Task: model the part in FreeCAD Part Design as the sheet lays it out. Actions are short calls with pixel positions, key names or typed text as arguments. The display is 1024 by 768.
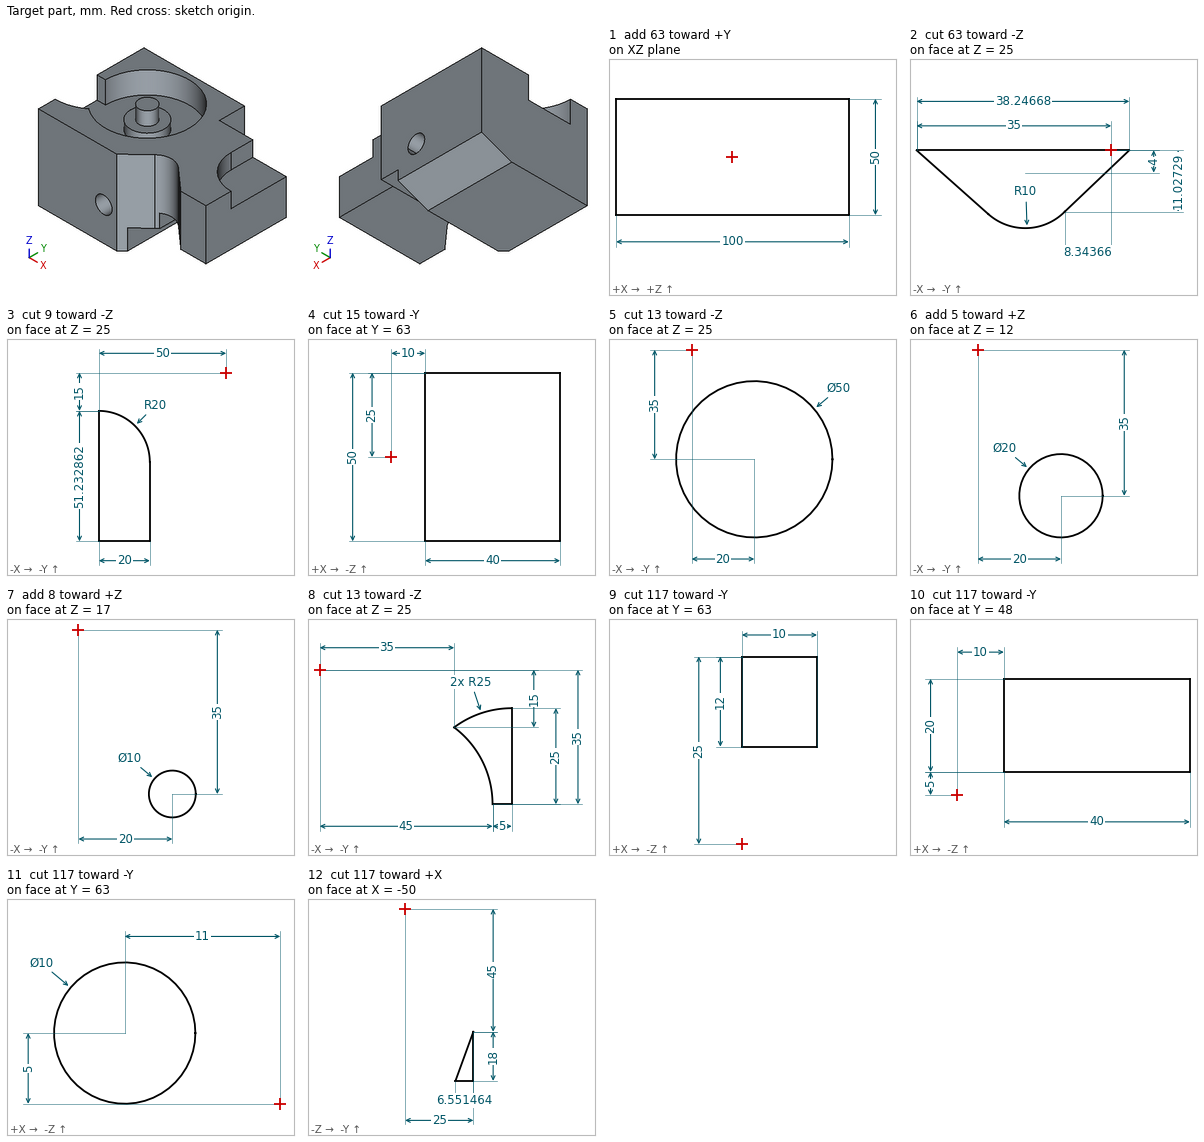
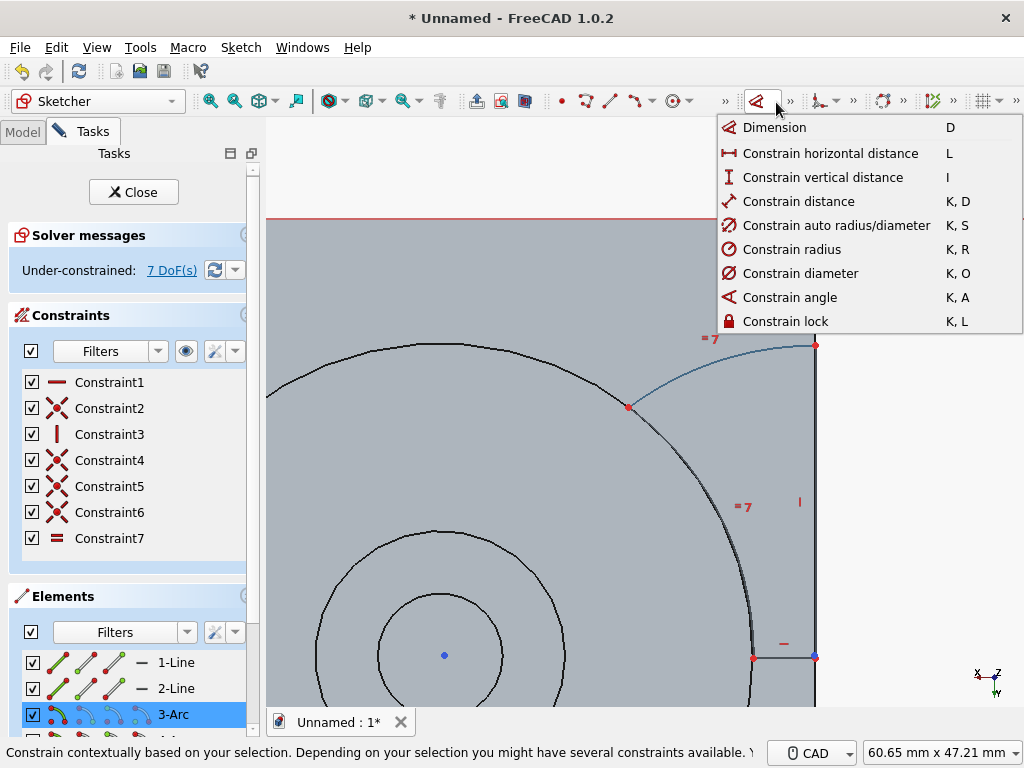
click(870, 249)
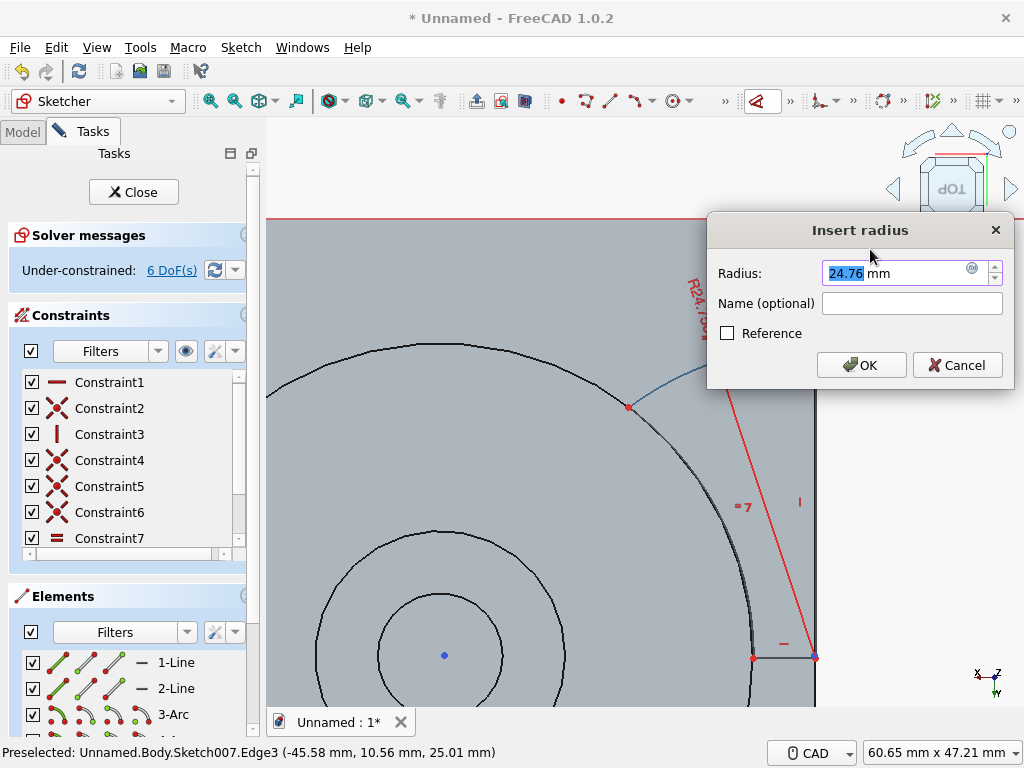
text(25)
key(Return)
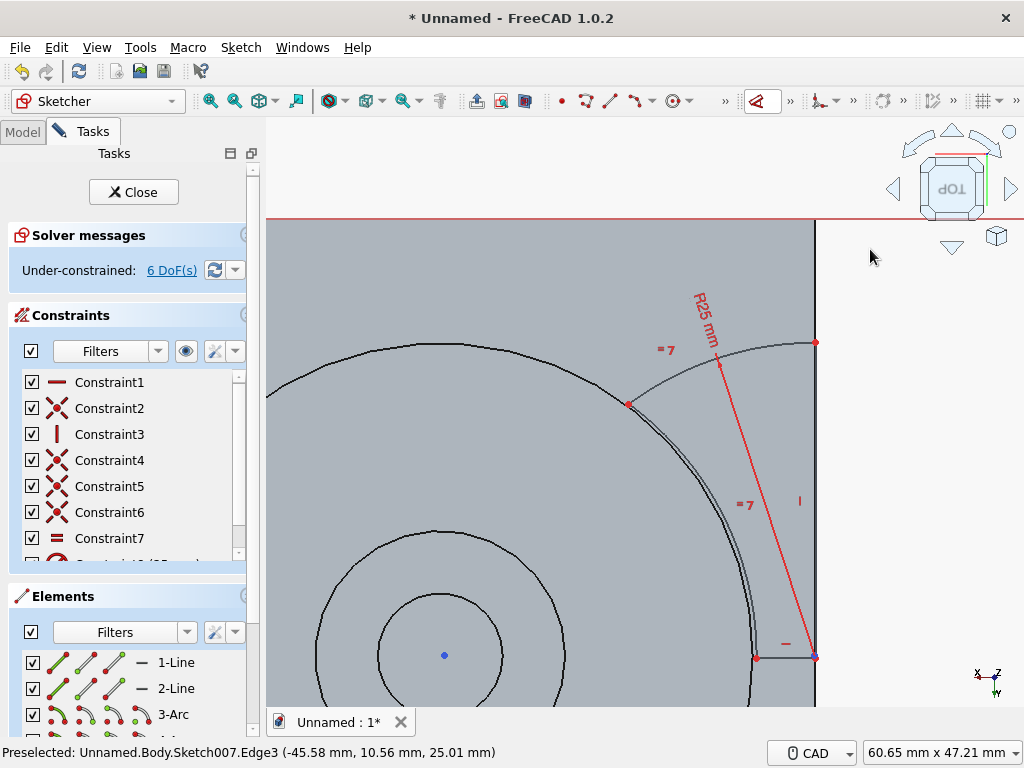
click(774, 658)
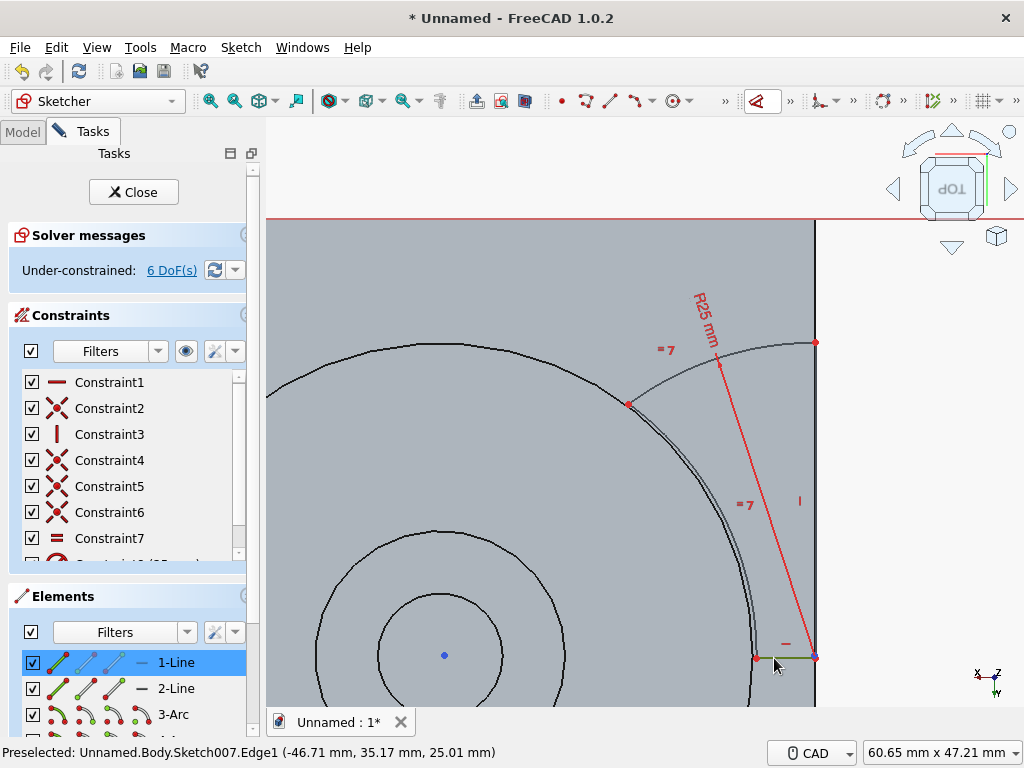
key(l)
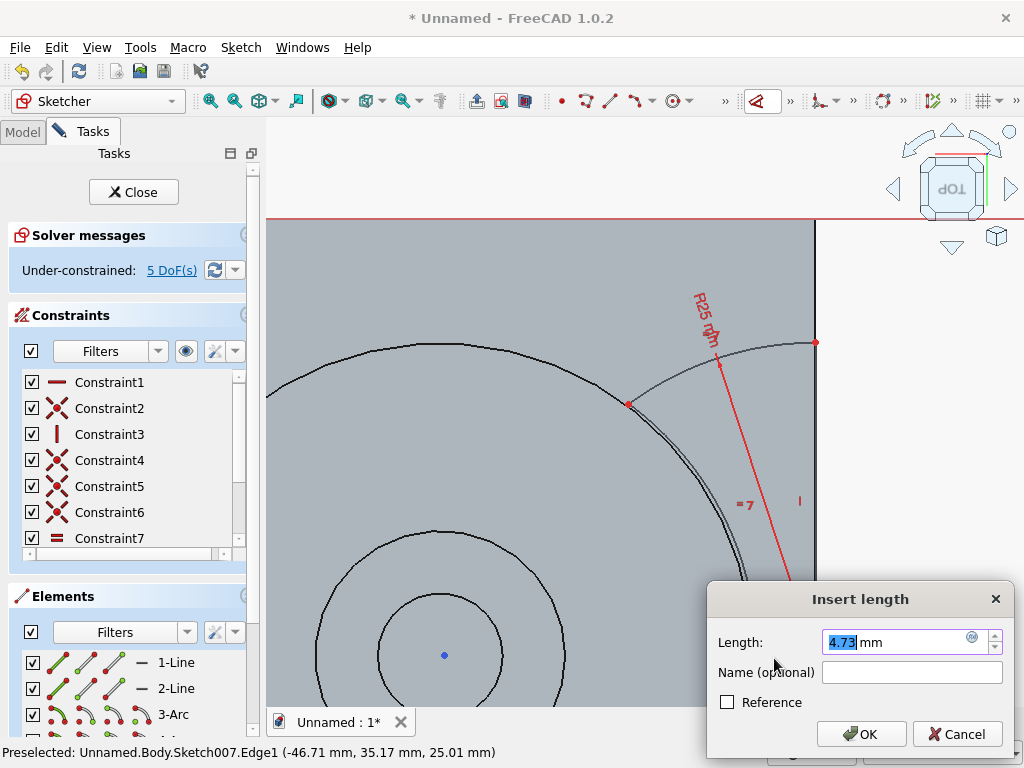
text(5)
key(Return)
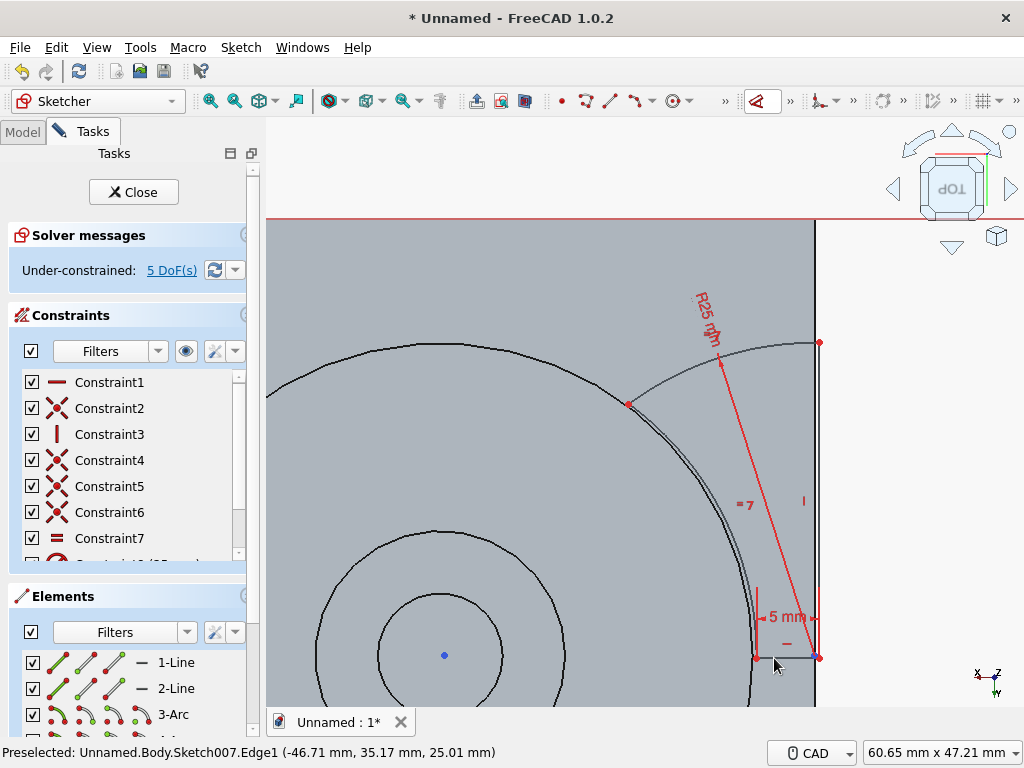
click(819, 564)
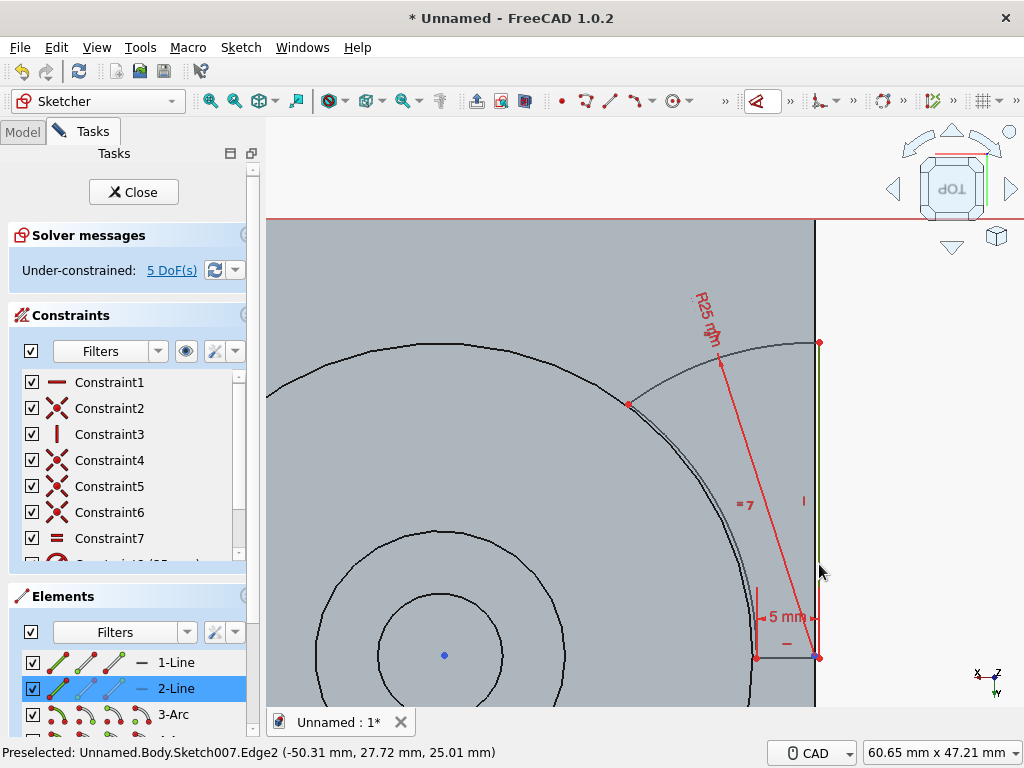
click(776, 102)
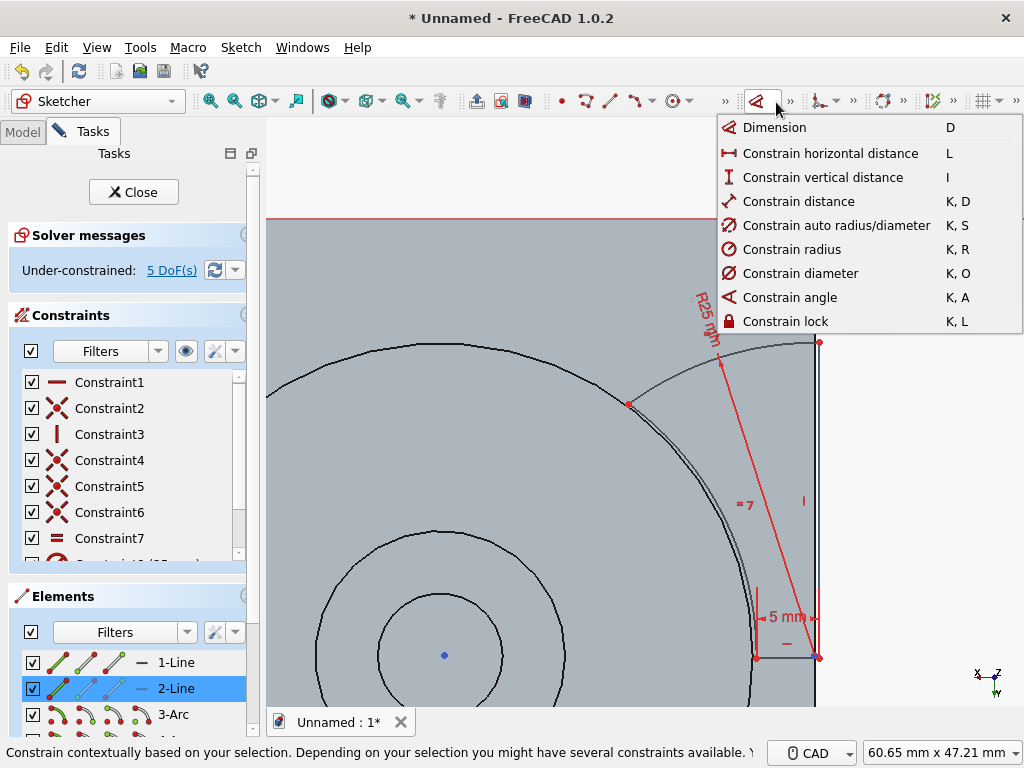
click(870, 177)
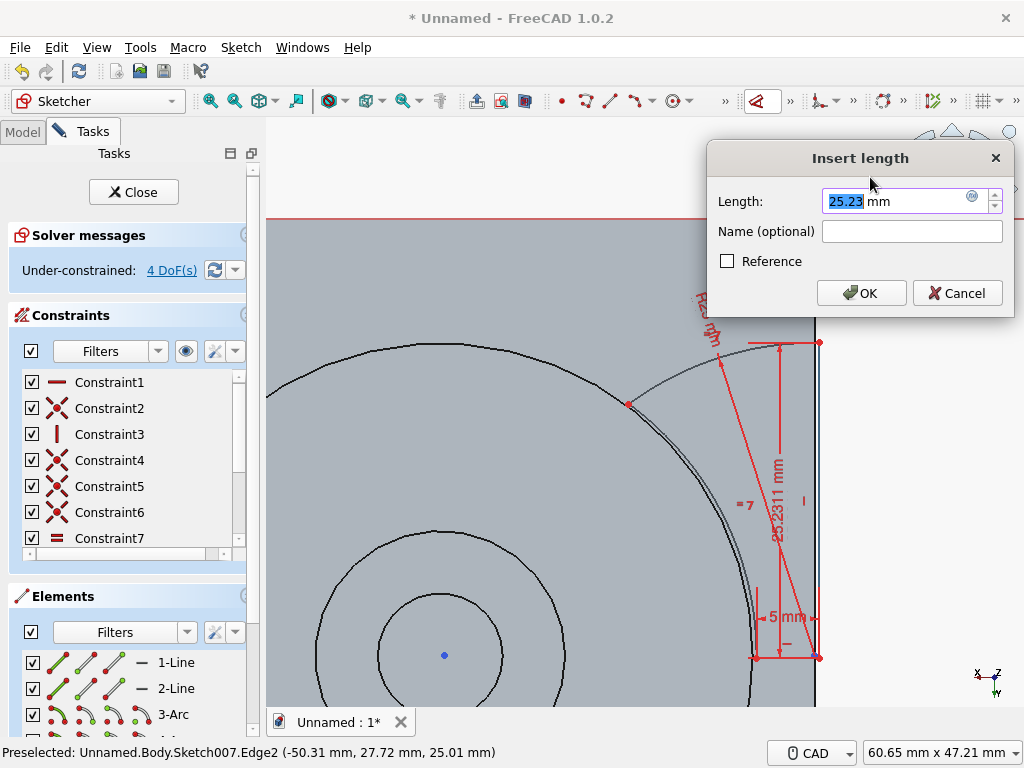
text(25)
key(Return)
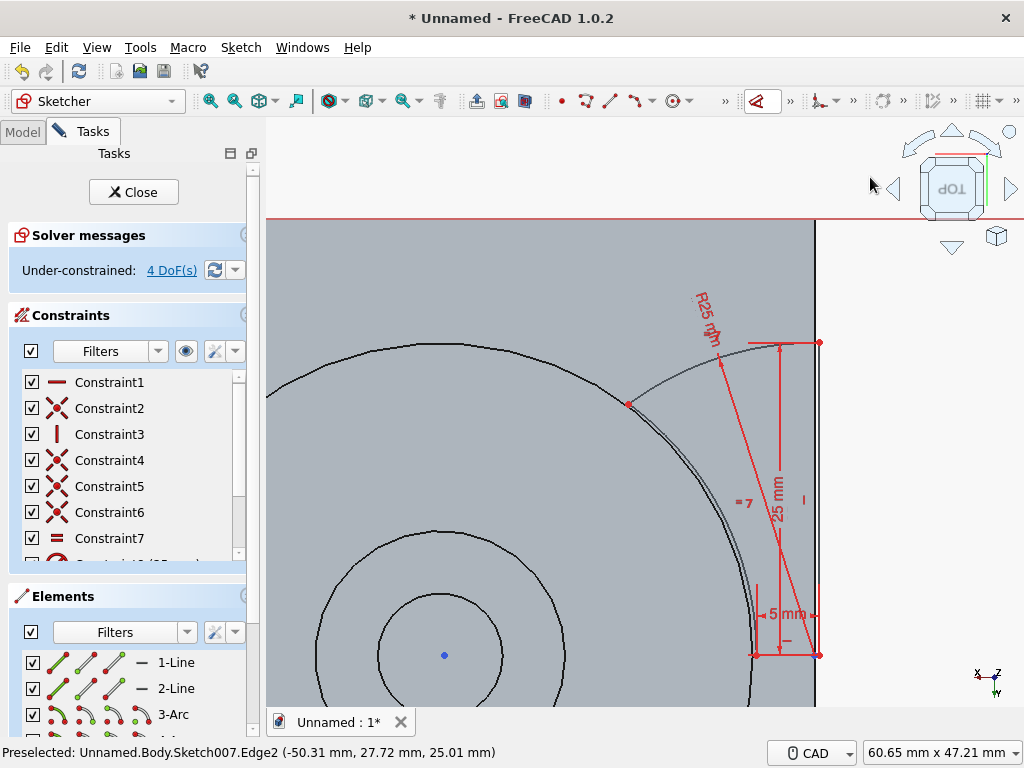
click(757, 655)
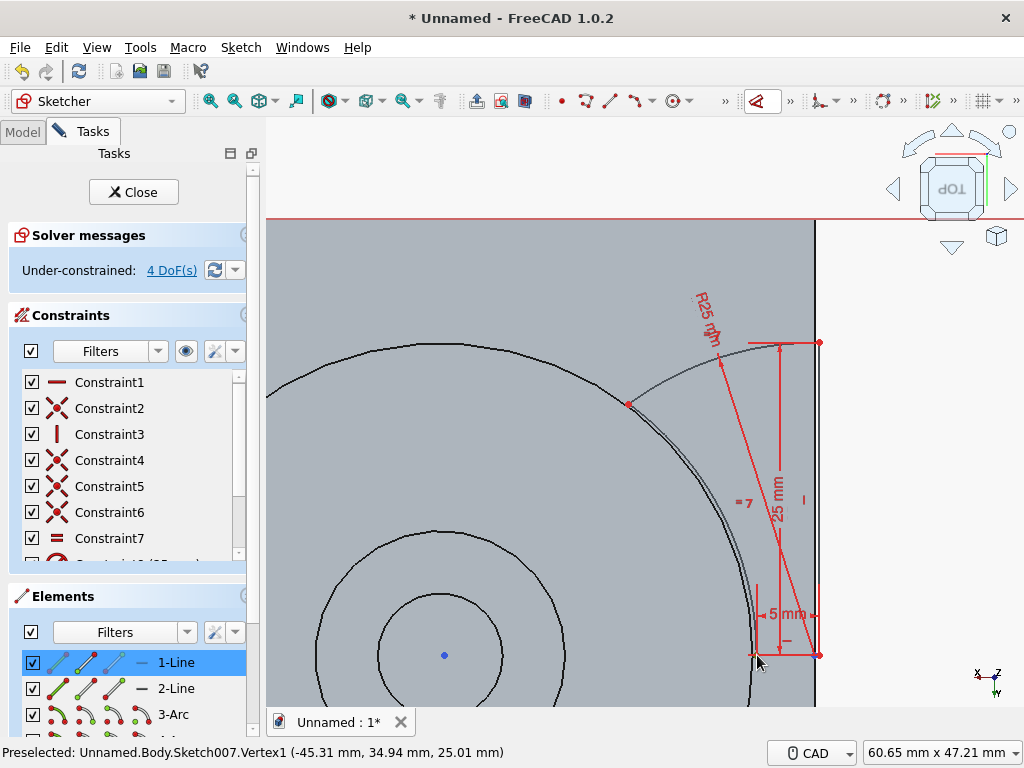
click(776, 102)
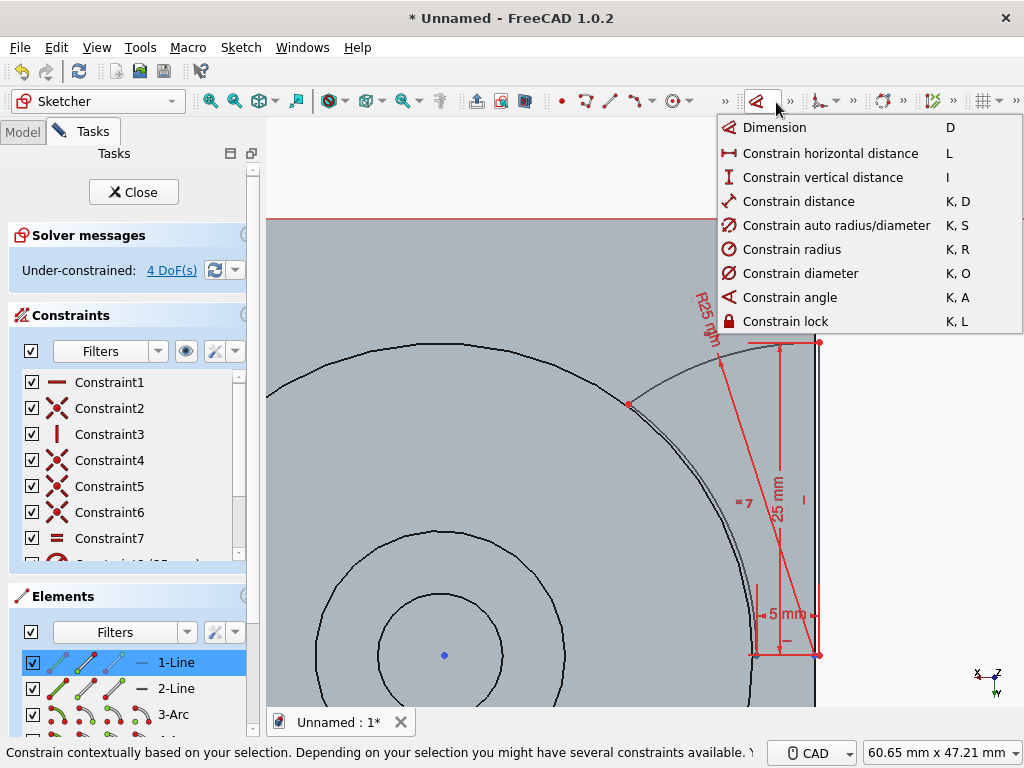
click(870, 153)